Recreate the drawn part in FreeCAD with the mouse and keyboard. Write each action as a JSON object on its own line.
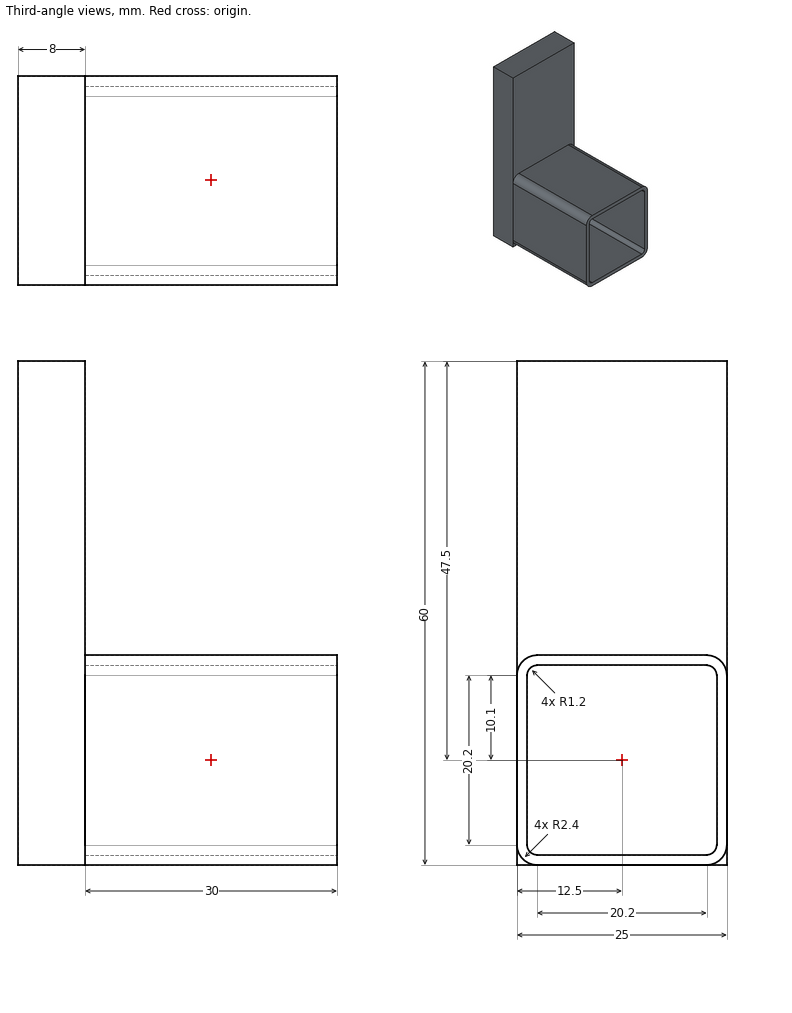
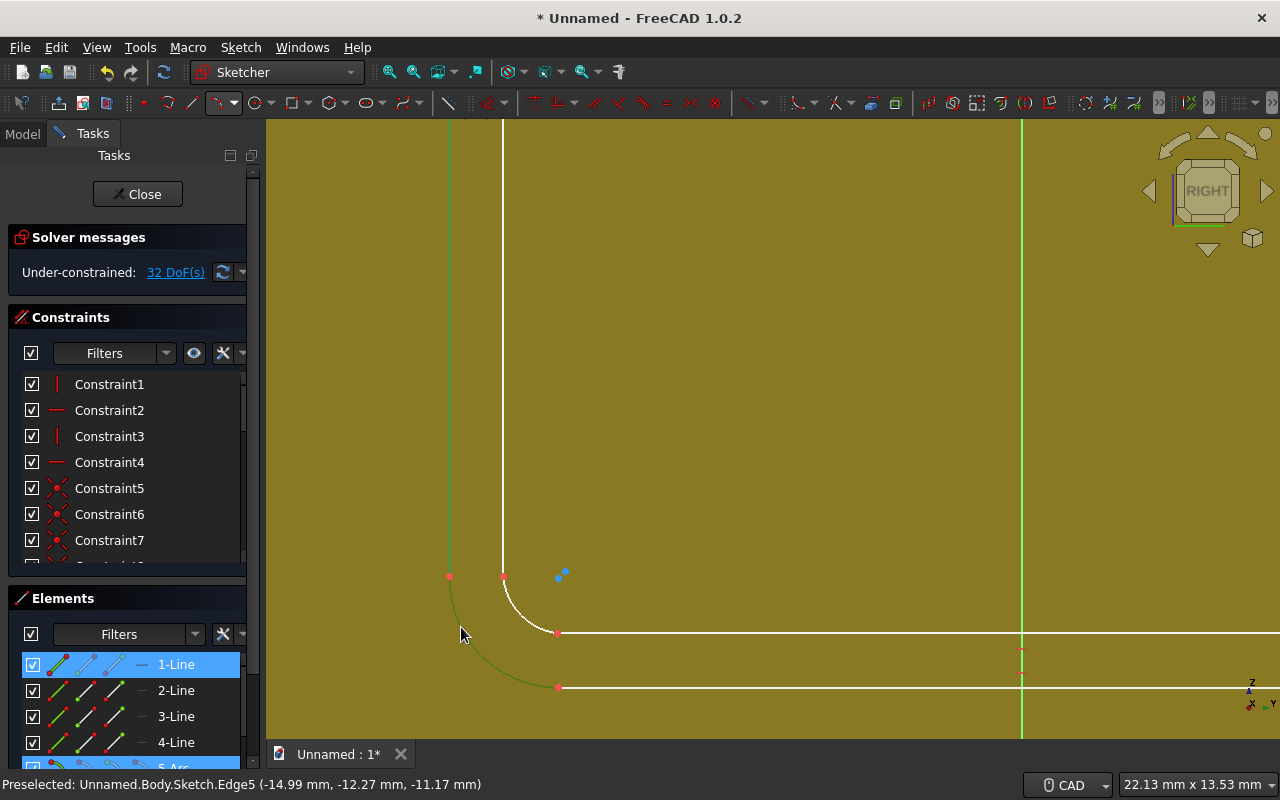
{"action": "key", "text": "t"}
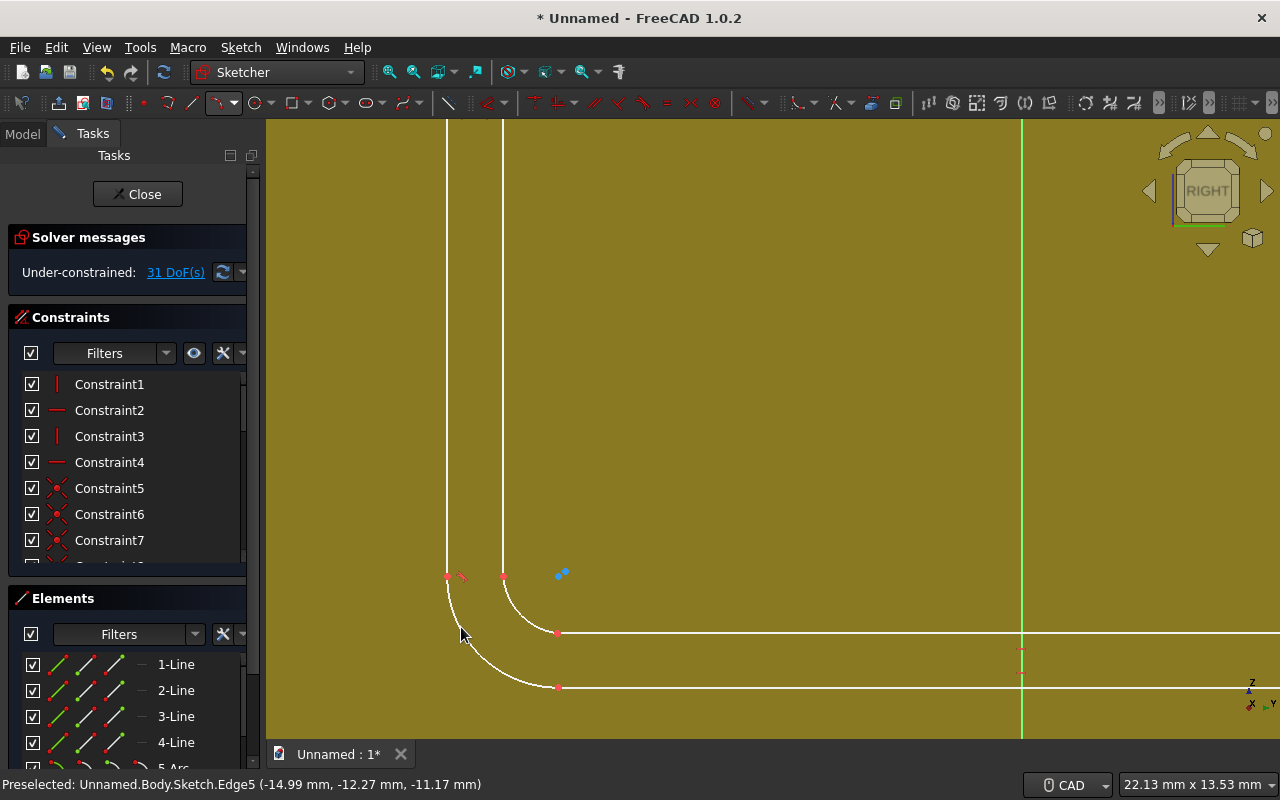
{"action": "left_click", "coordinate": [447, 299]}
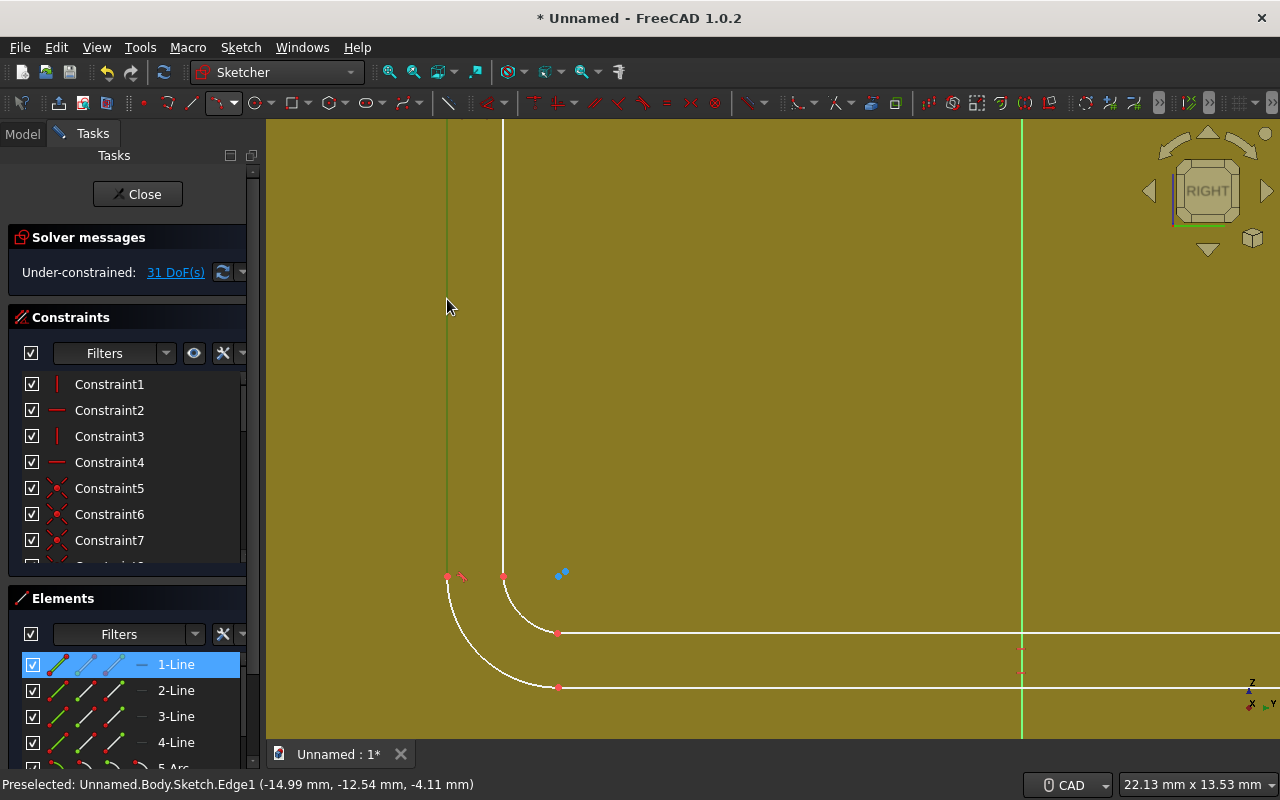
{"action": "scroll", "coordinate": [520, 614], "scroll_direction": "down", "scroll_amount": 5}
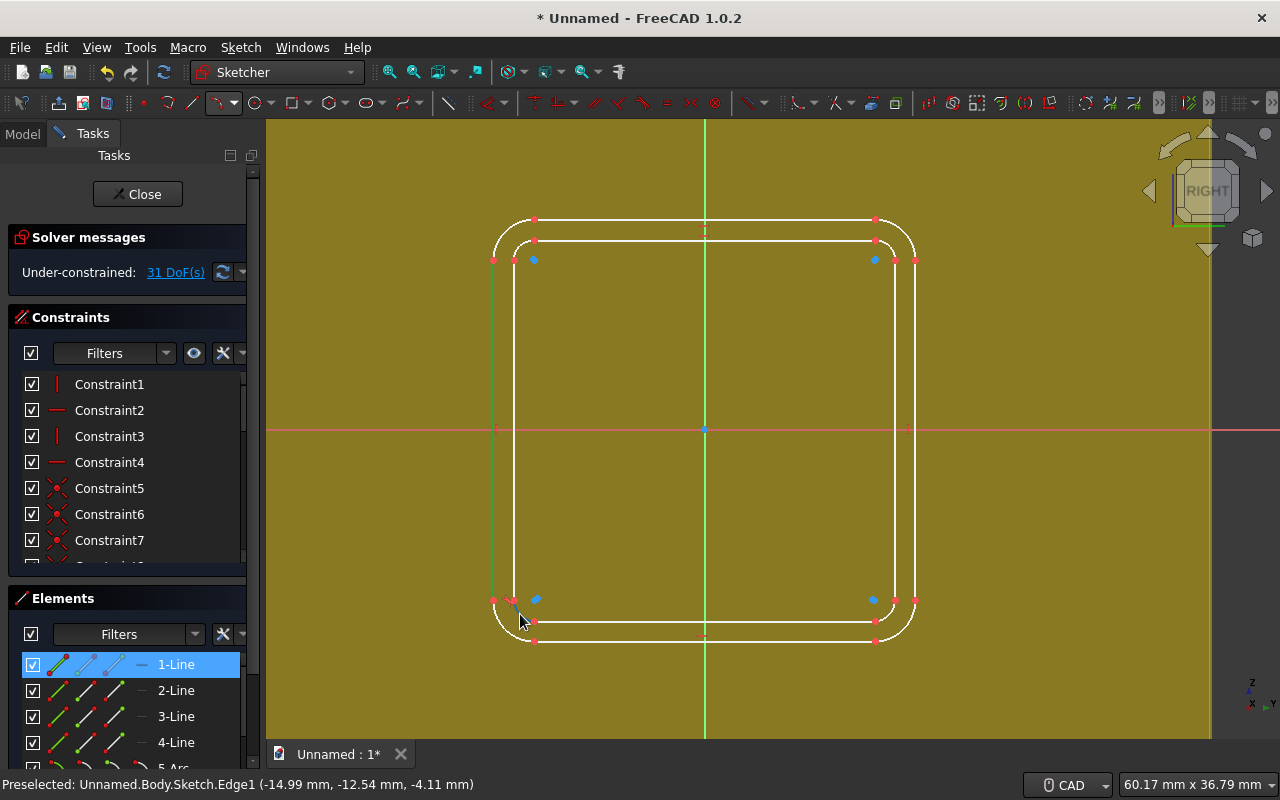
{"action": "left_click", "coordinate": [516, 224]}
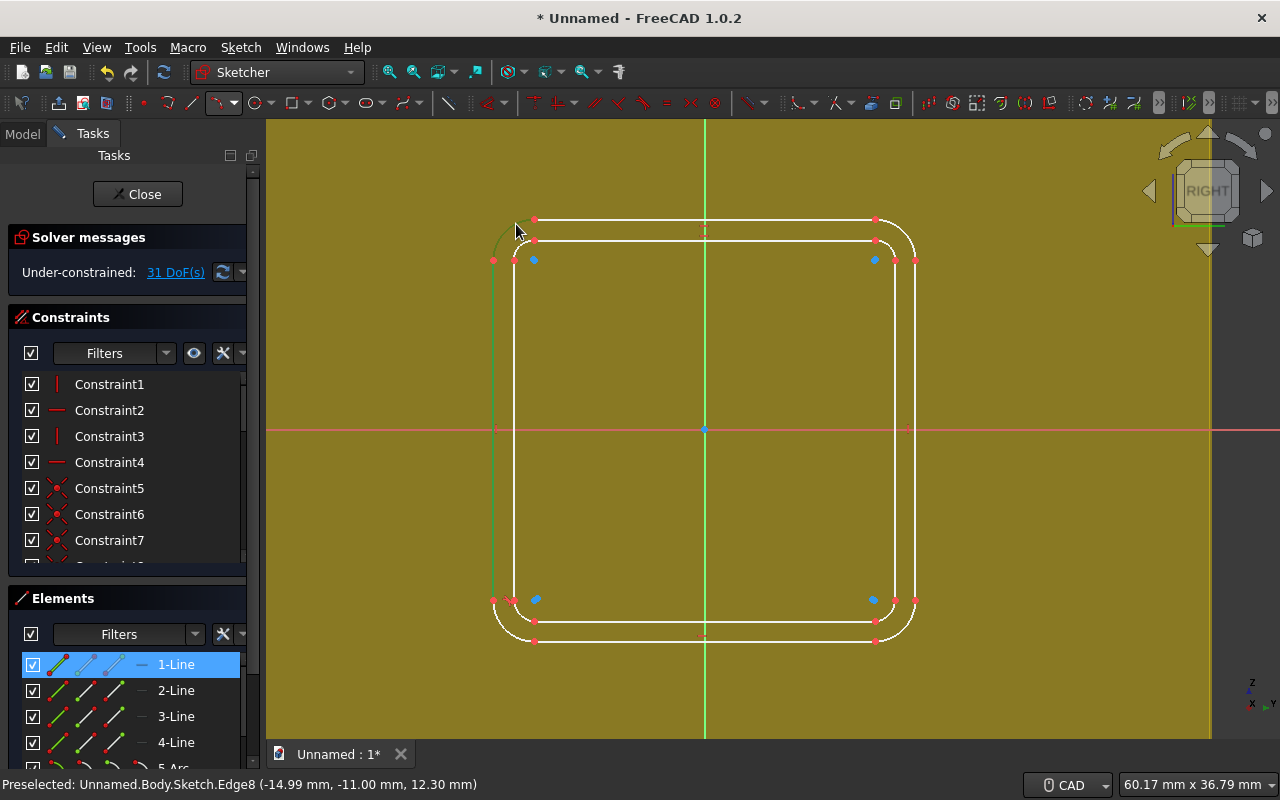
{"action": "key", "text": "t"}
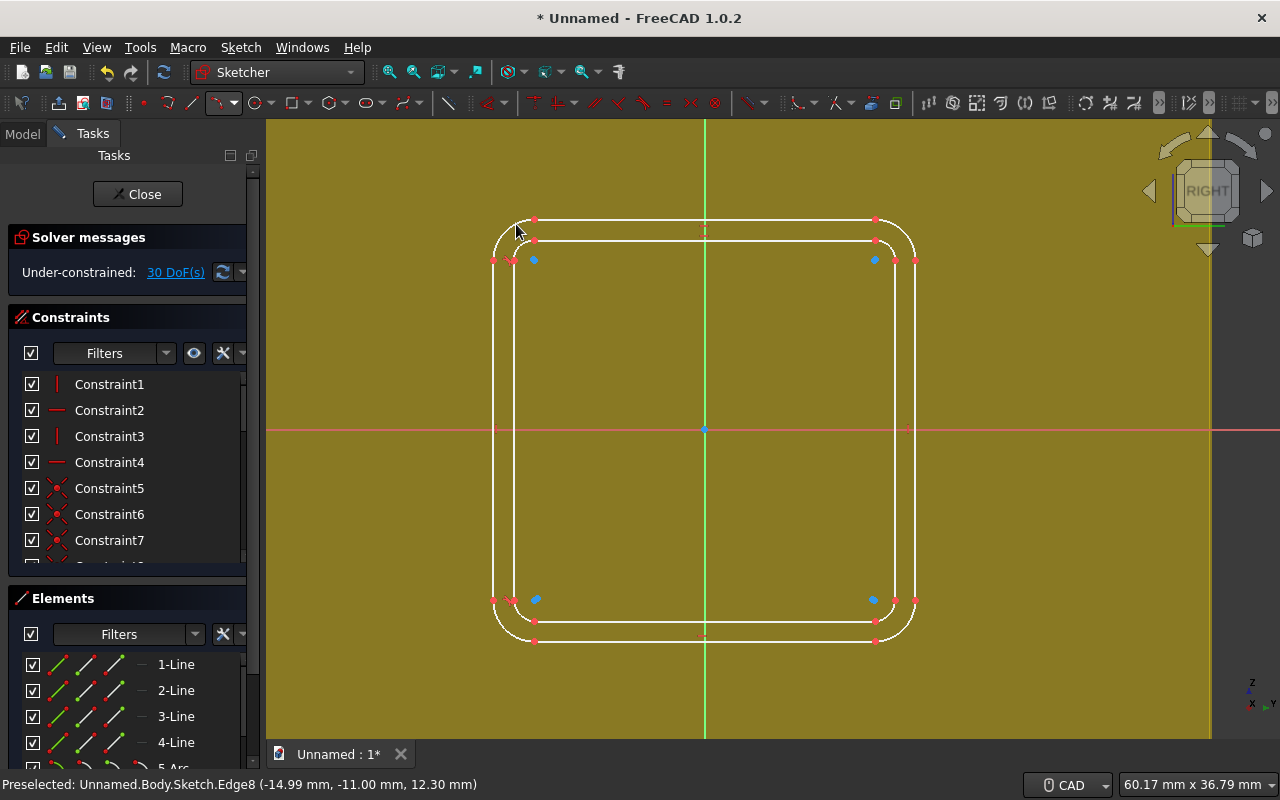
{"action": "left_click", "coordinate": [637, 642]}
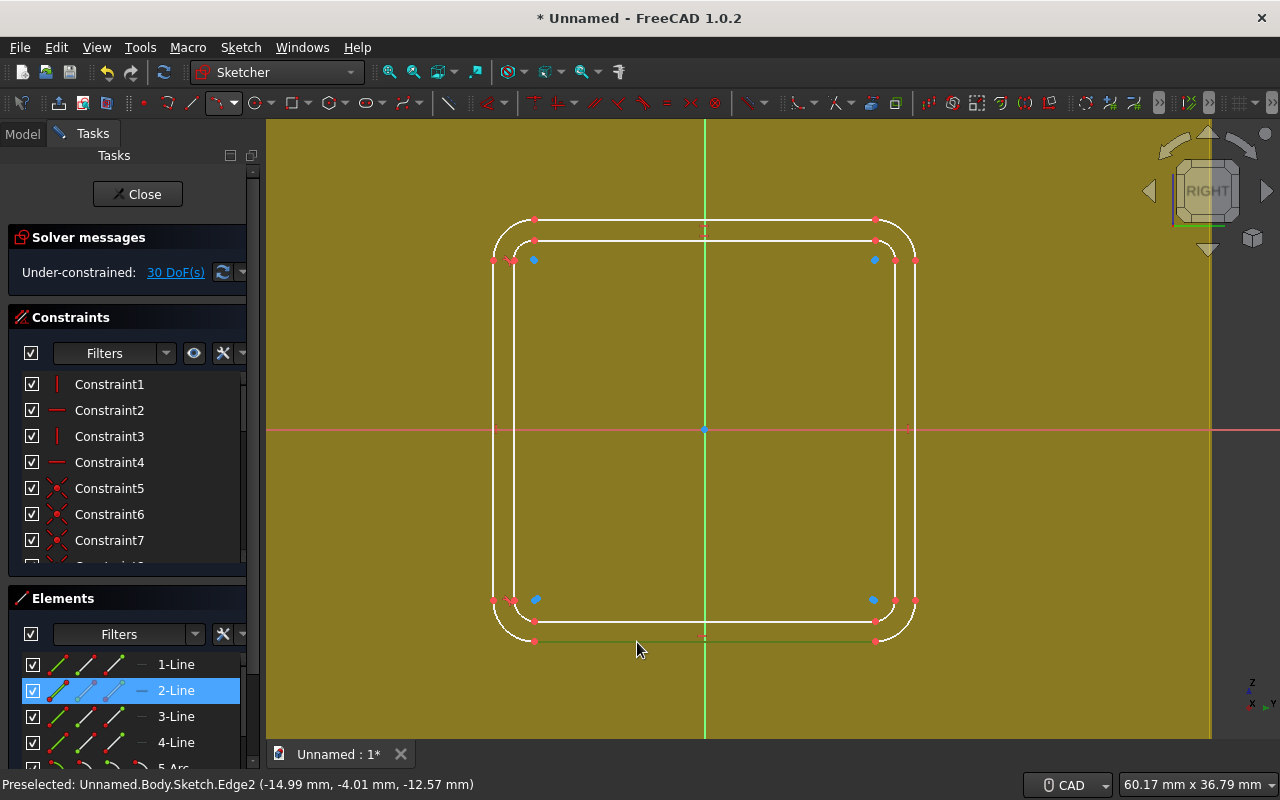
{"action": "left_click", "coordinate": [498, 619]}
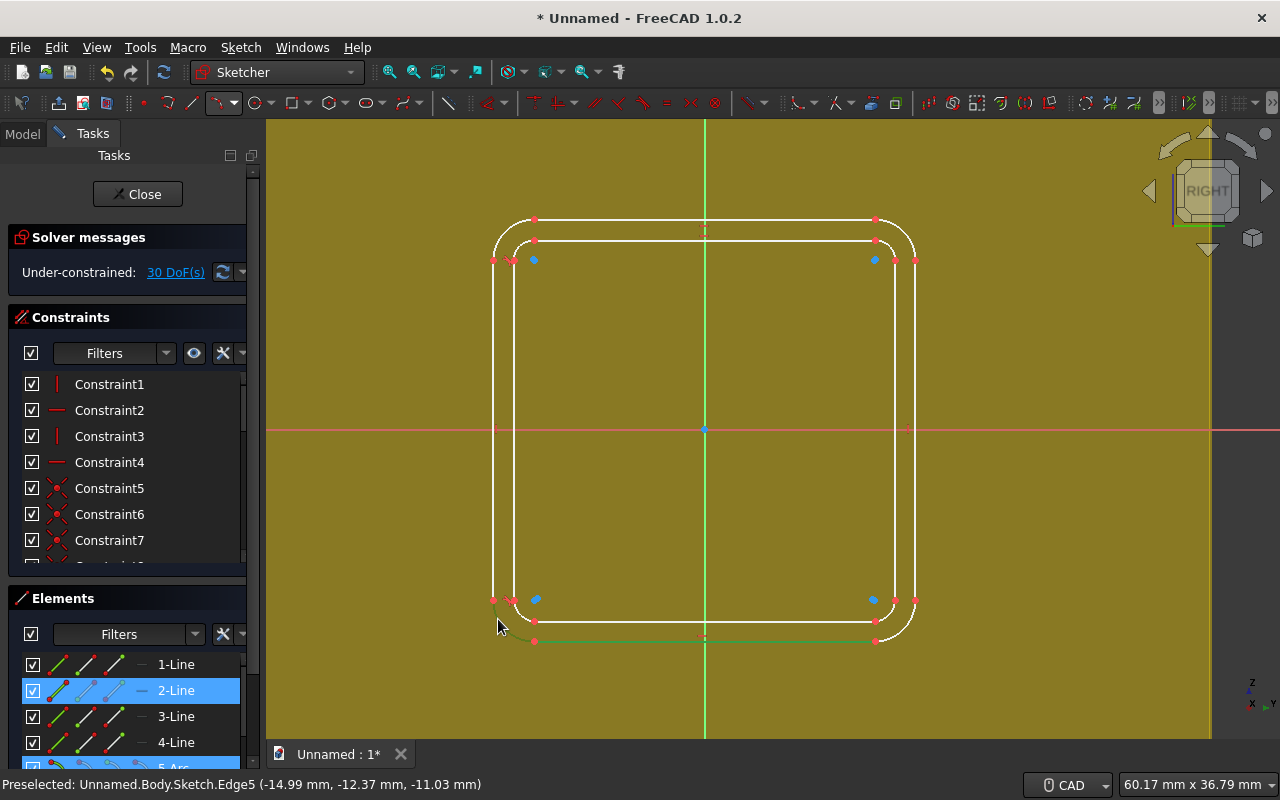
{"action": "key", "text": "t"}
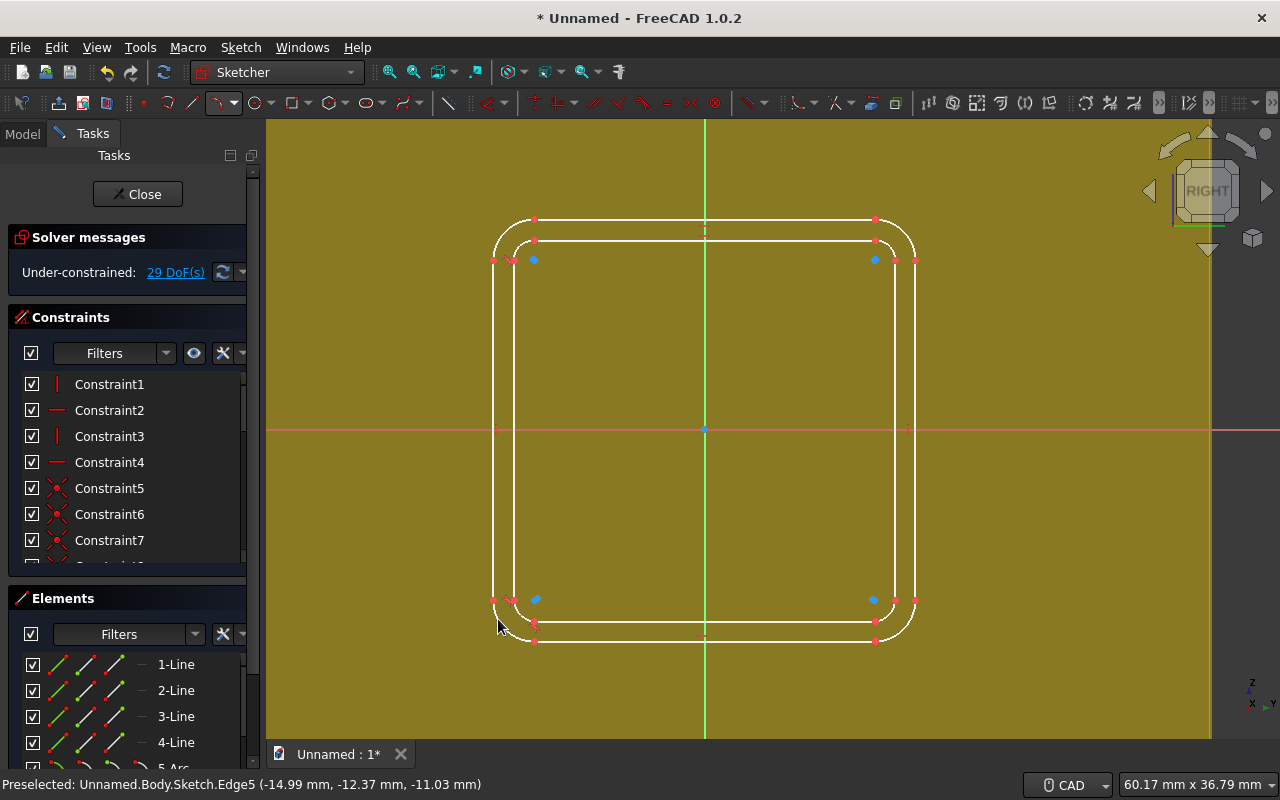
{"action": "left_click", "coordinate": [637, 642]}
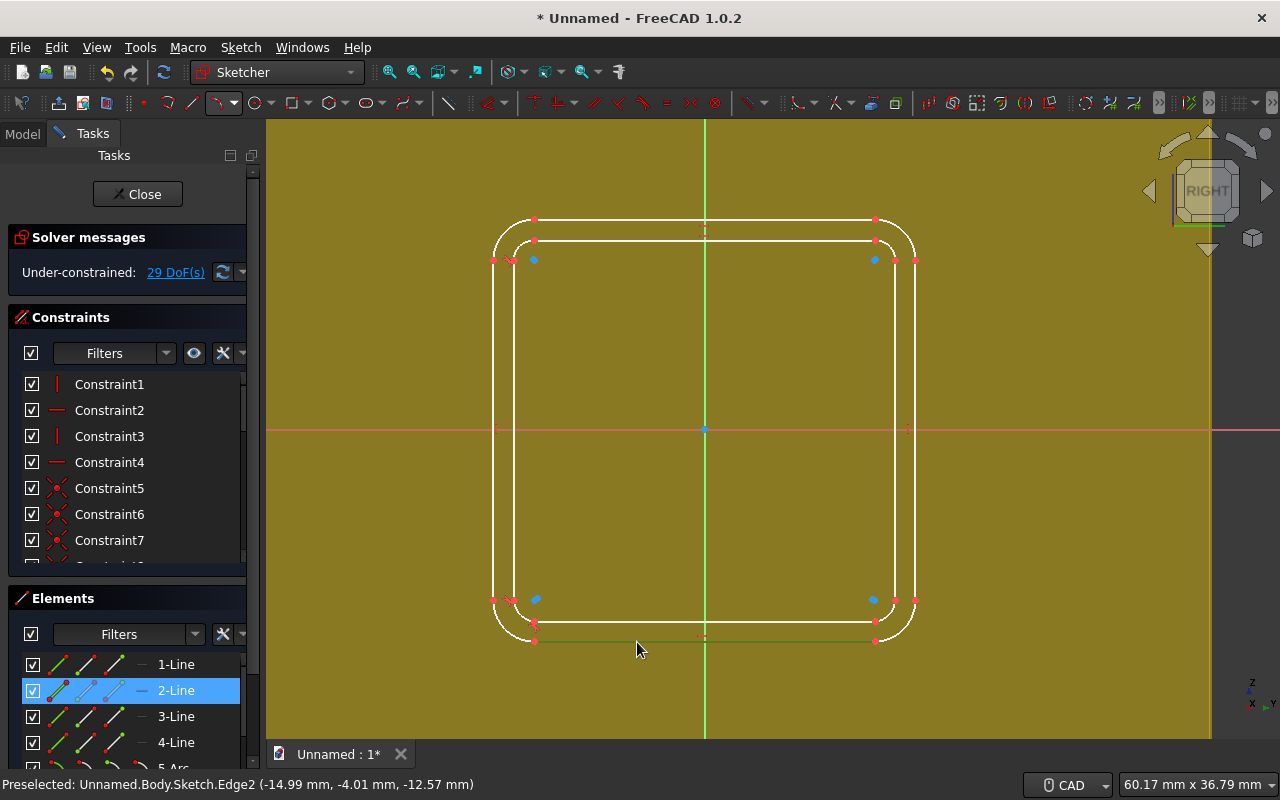
{"action": "left_click", "coordinate": [894, 637]}